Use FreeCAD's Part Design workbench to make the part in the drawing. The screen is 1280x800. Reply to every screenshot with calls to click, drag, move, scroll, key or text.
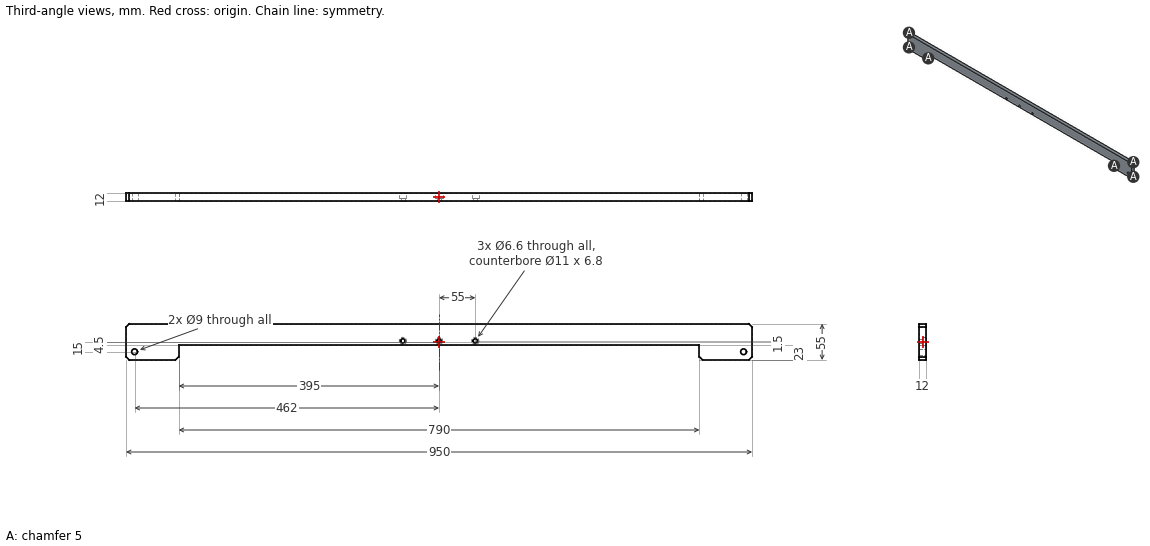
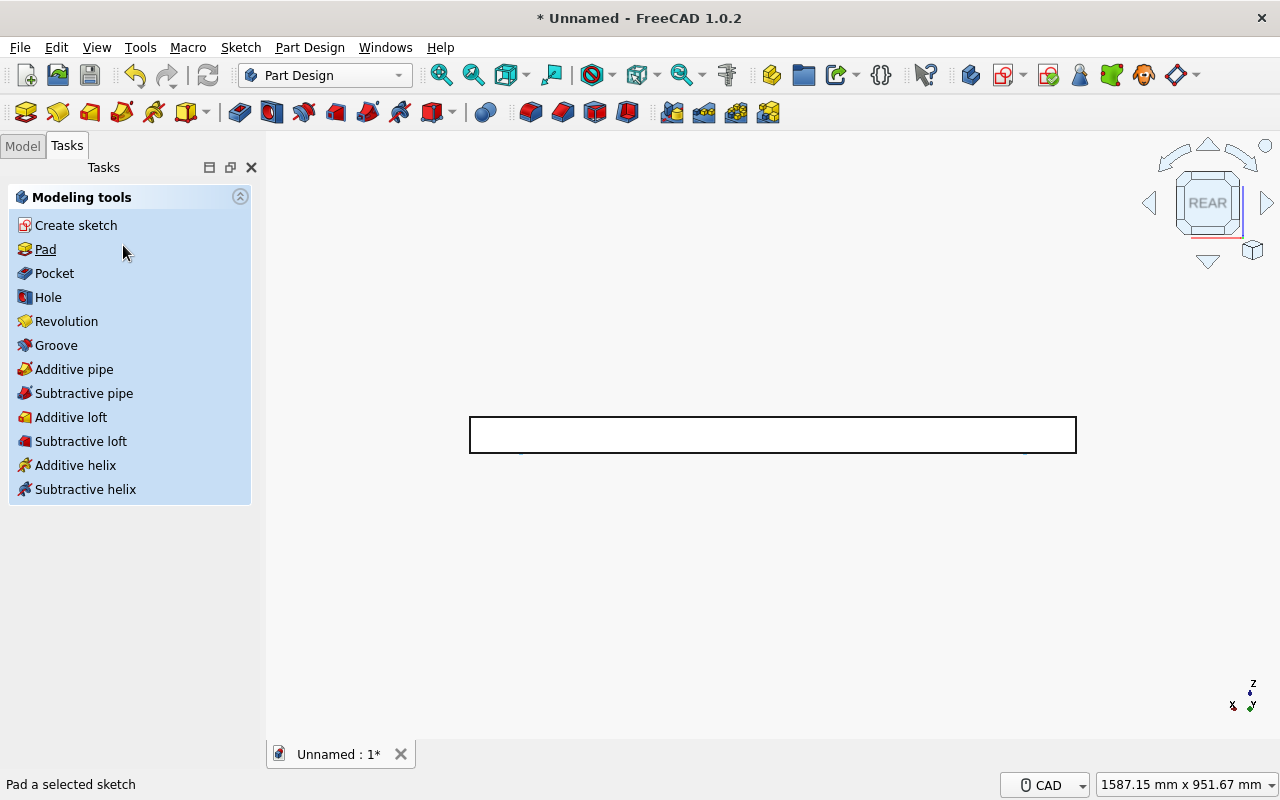
click(240, 112)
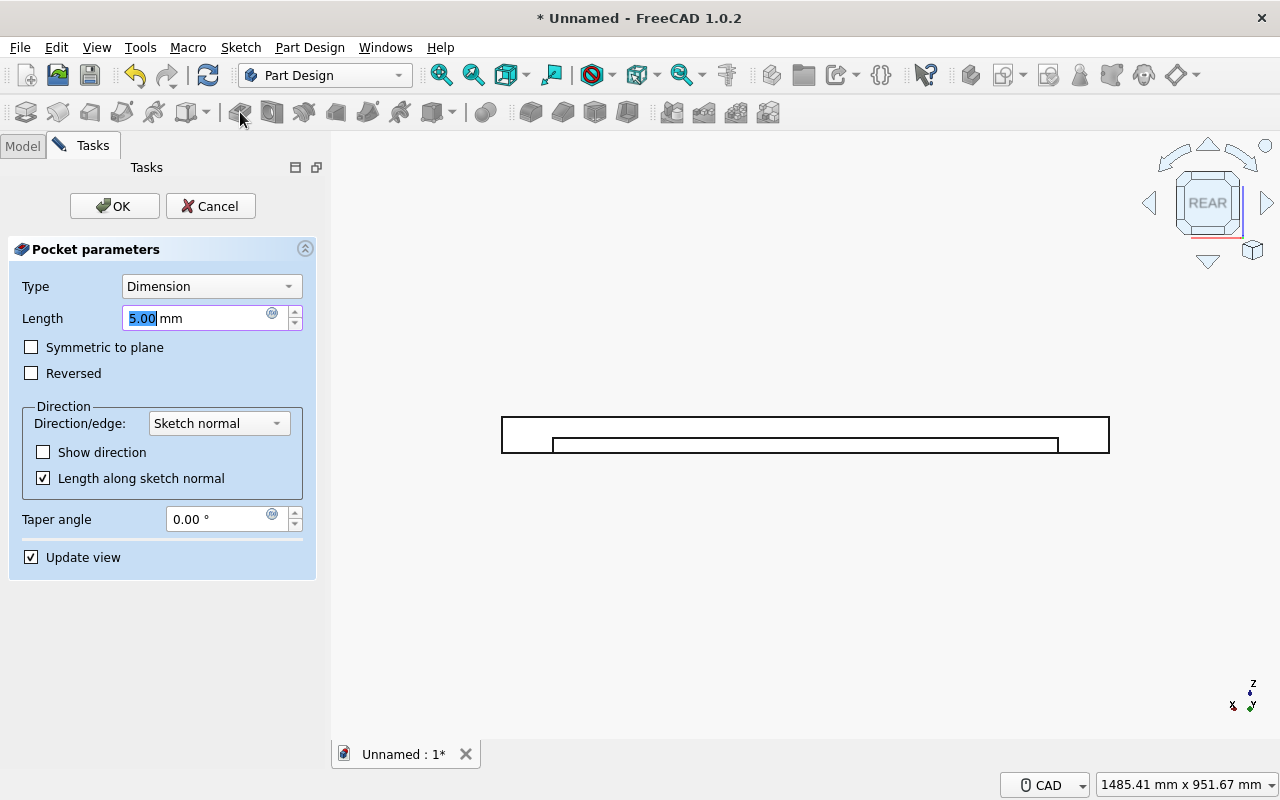
text(12)
key(Tab)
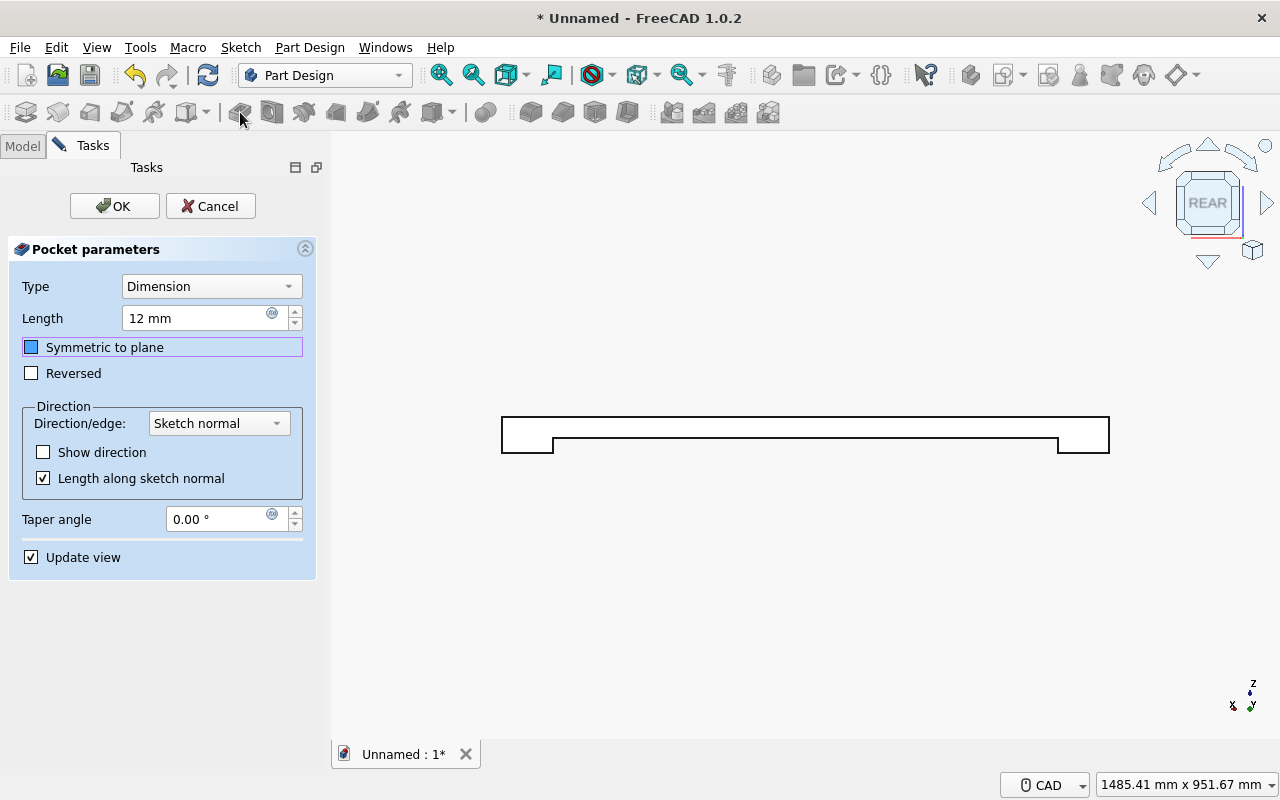
click(115, 206)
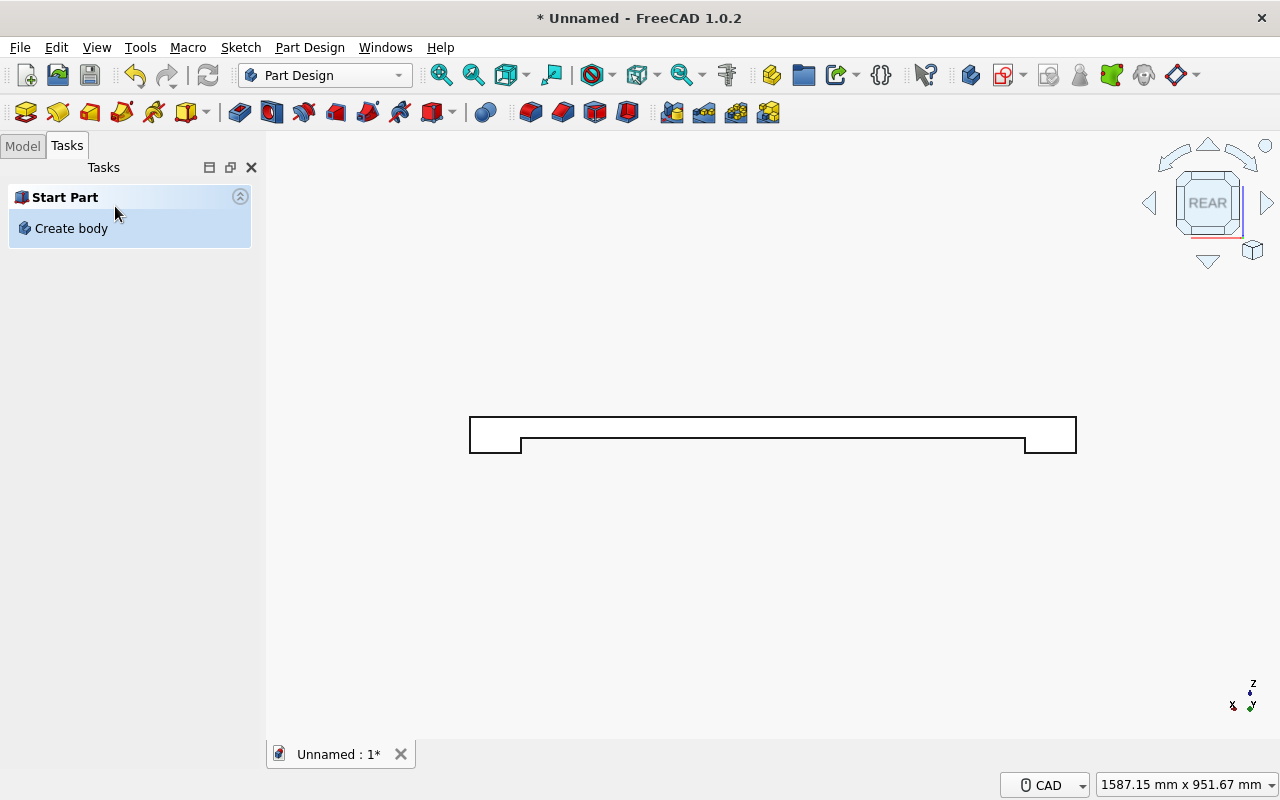
scroll(1025, 452, up, 9)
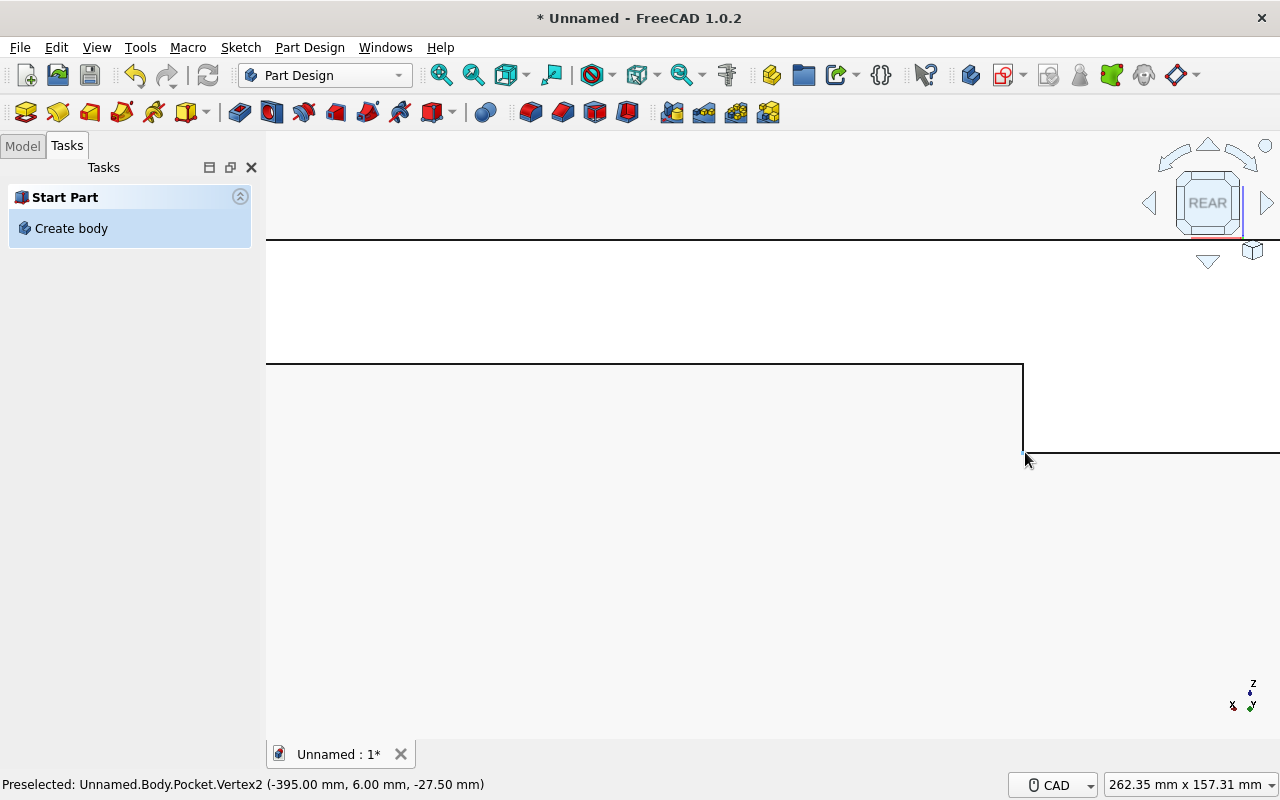
key(v)
key(f)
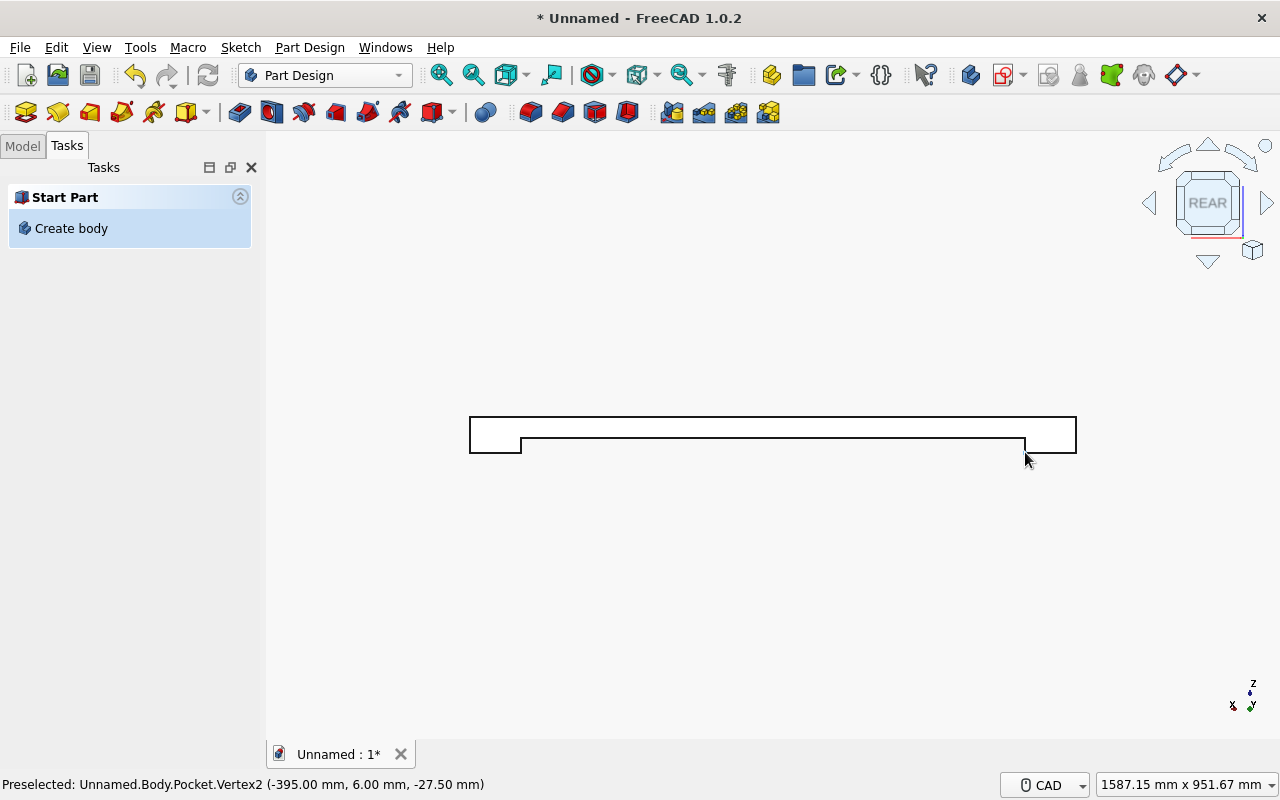
key(0)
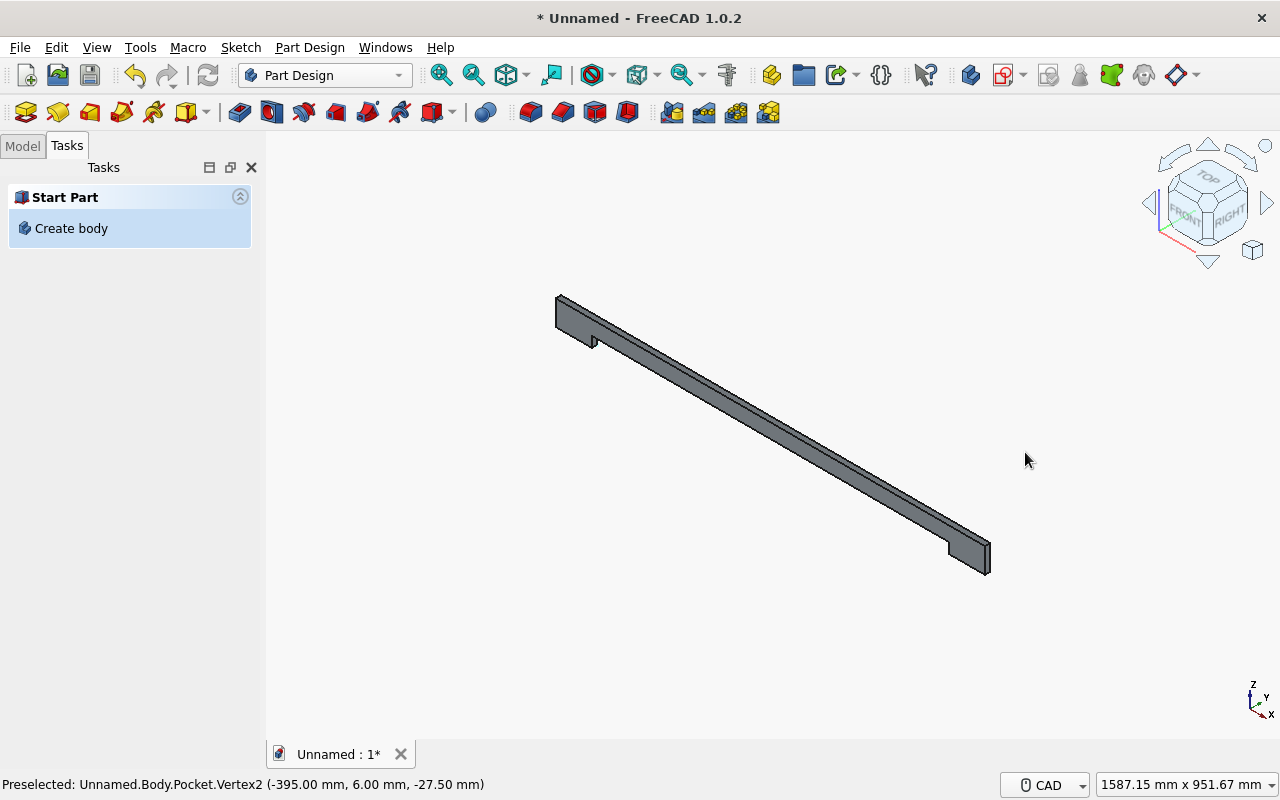
scroll(595, 345, up, 9)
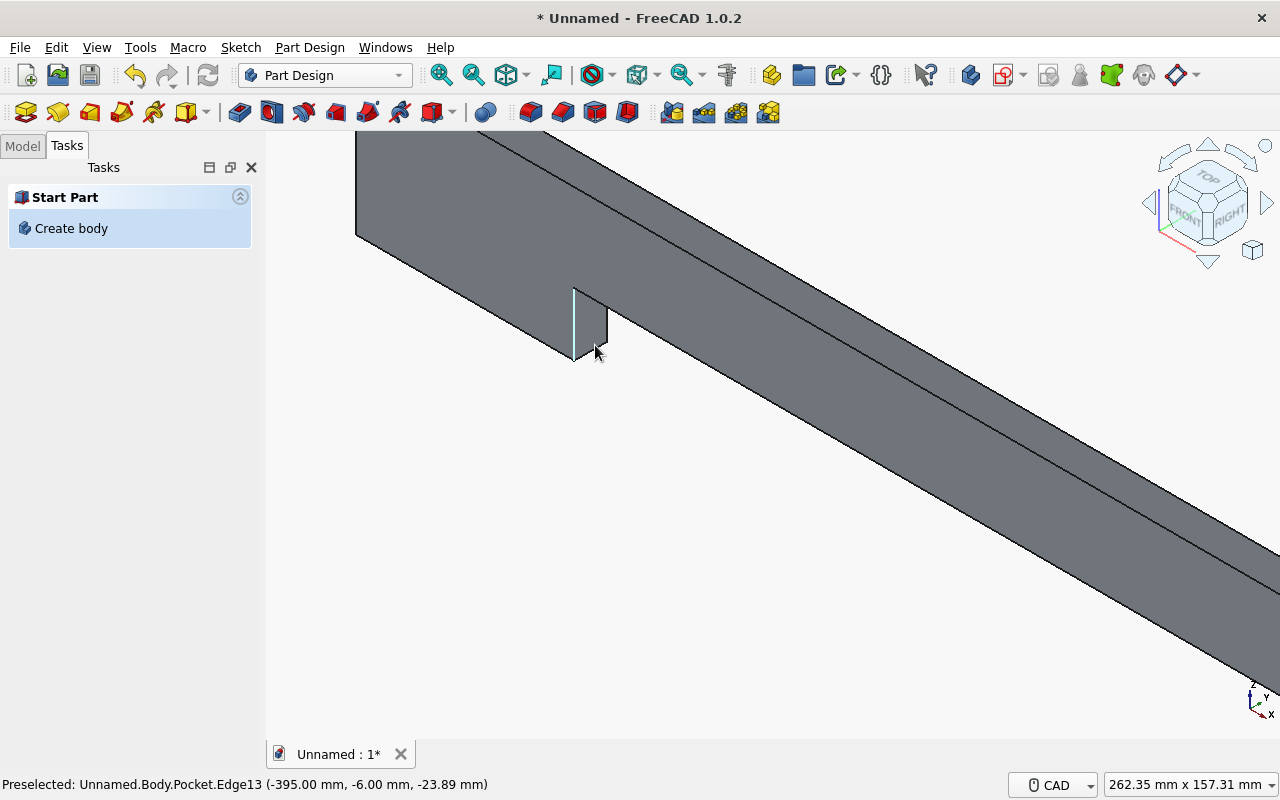
key(v)
key(f)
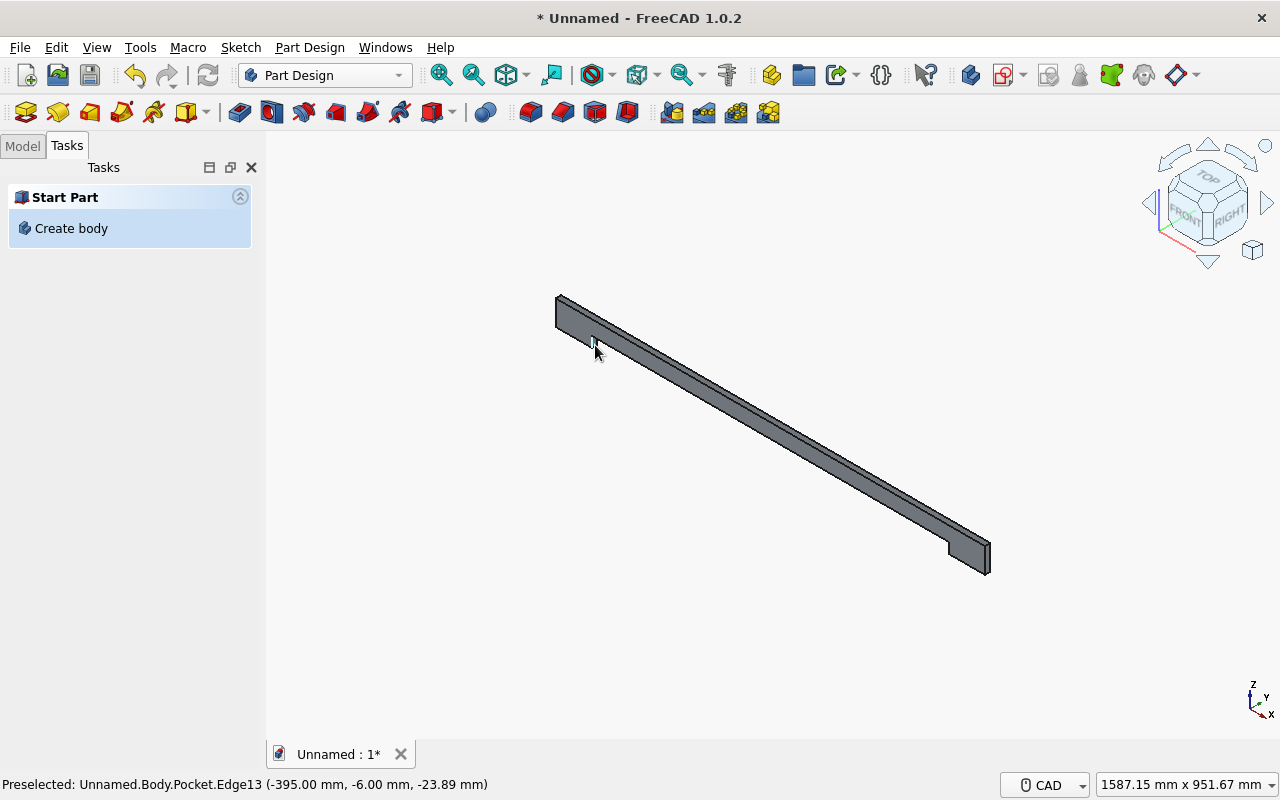
key(2)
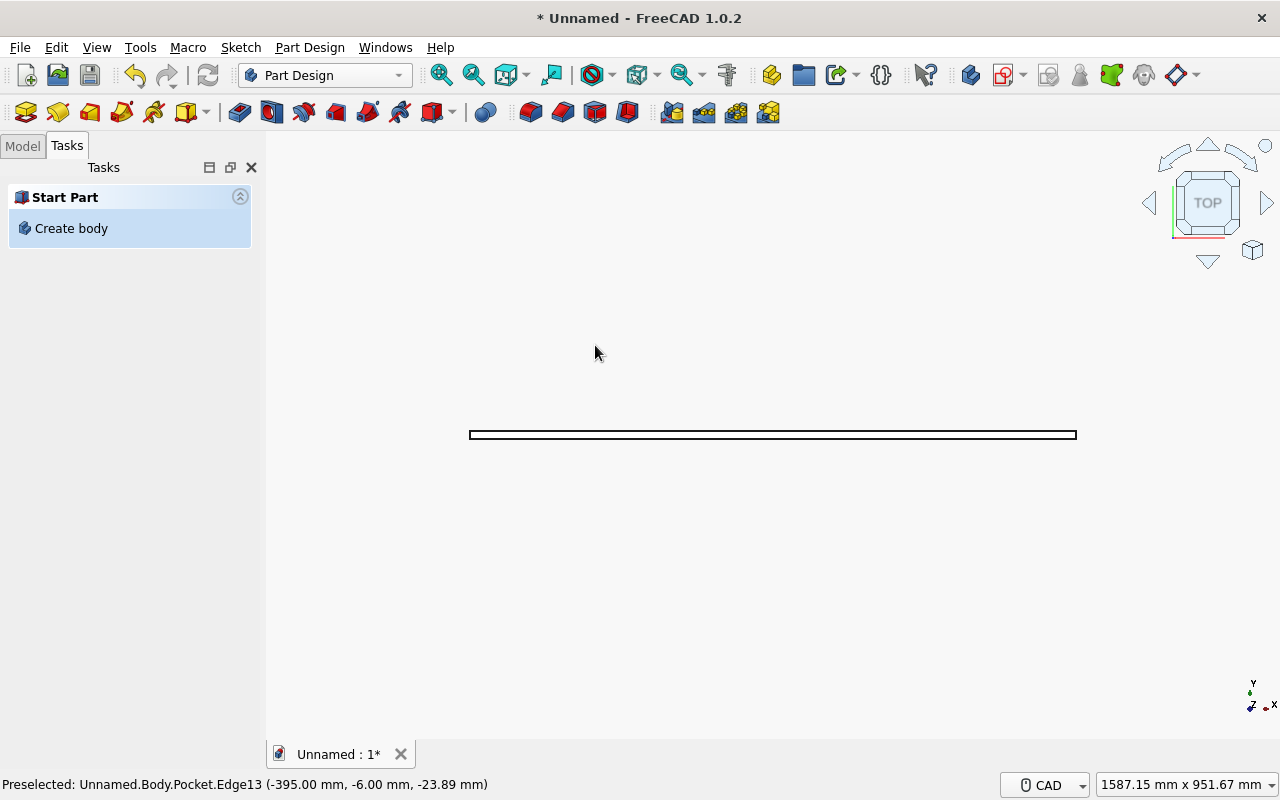
scroll(521, 434, up, 9)